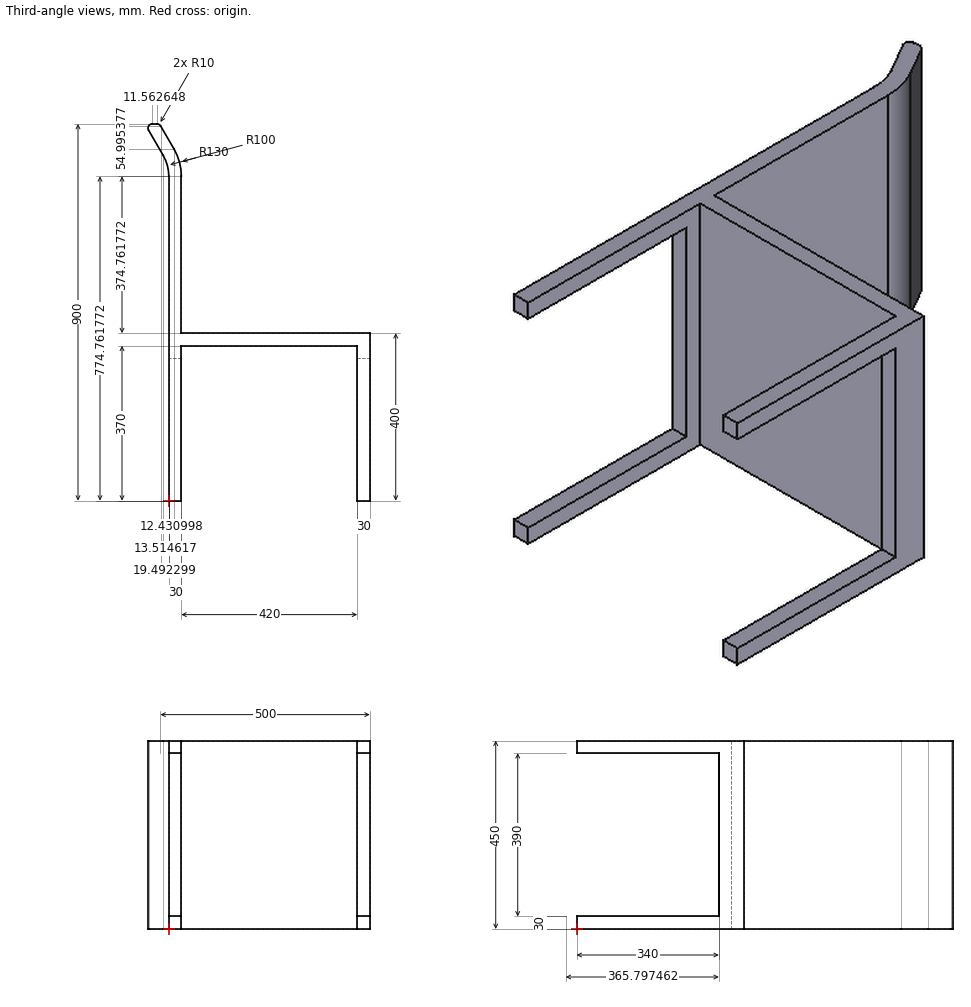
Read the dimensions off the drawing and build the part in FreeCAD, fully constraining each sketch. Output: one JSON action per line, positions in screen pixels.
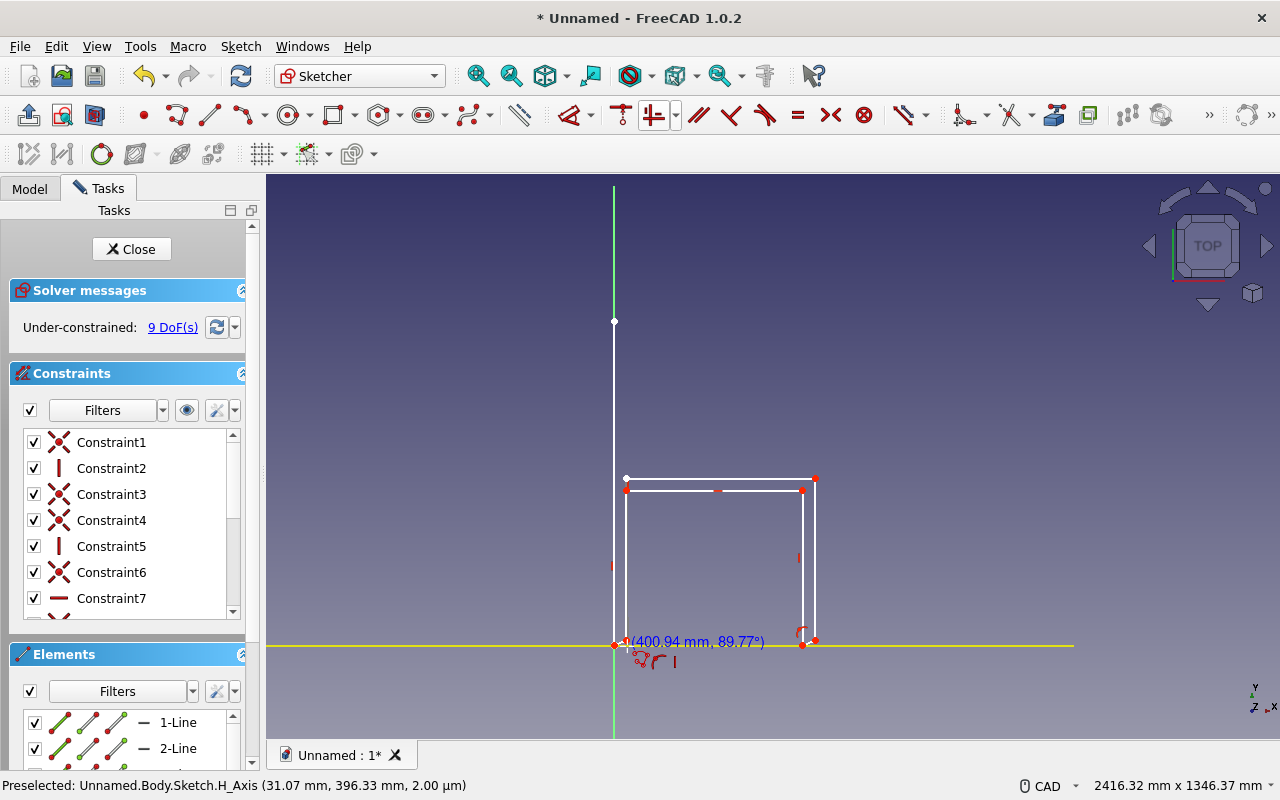
{"action": "scroll", "coordinate": [627, 321], "scroll_direction": "up", "scroll_amount": 2}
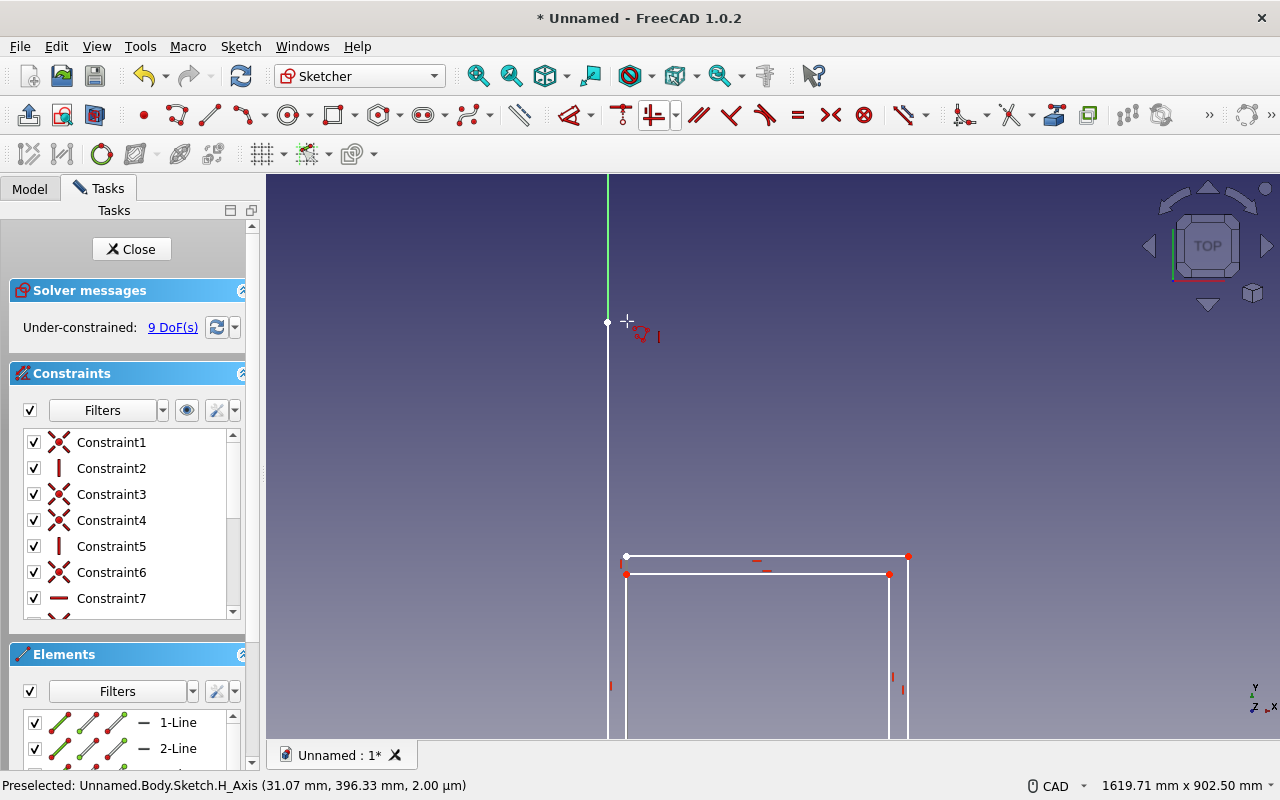
{"action": "left_click", "coordinate": [626, 320]}
{"action": "right_click", "coordinate": [626, 320]}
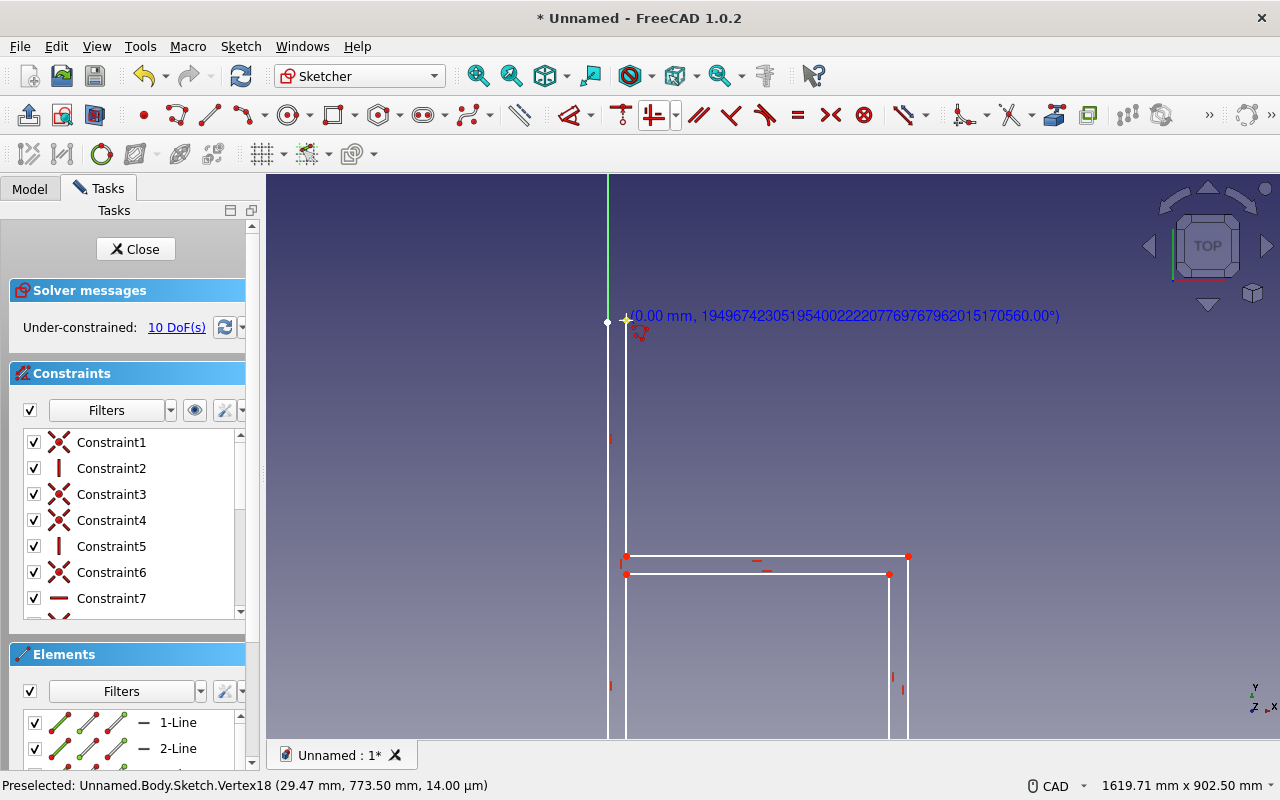
{"action": "key", "text": "g l"}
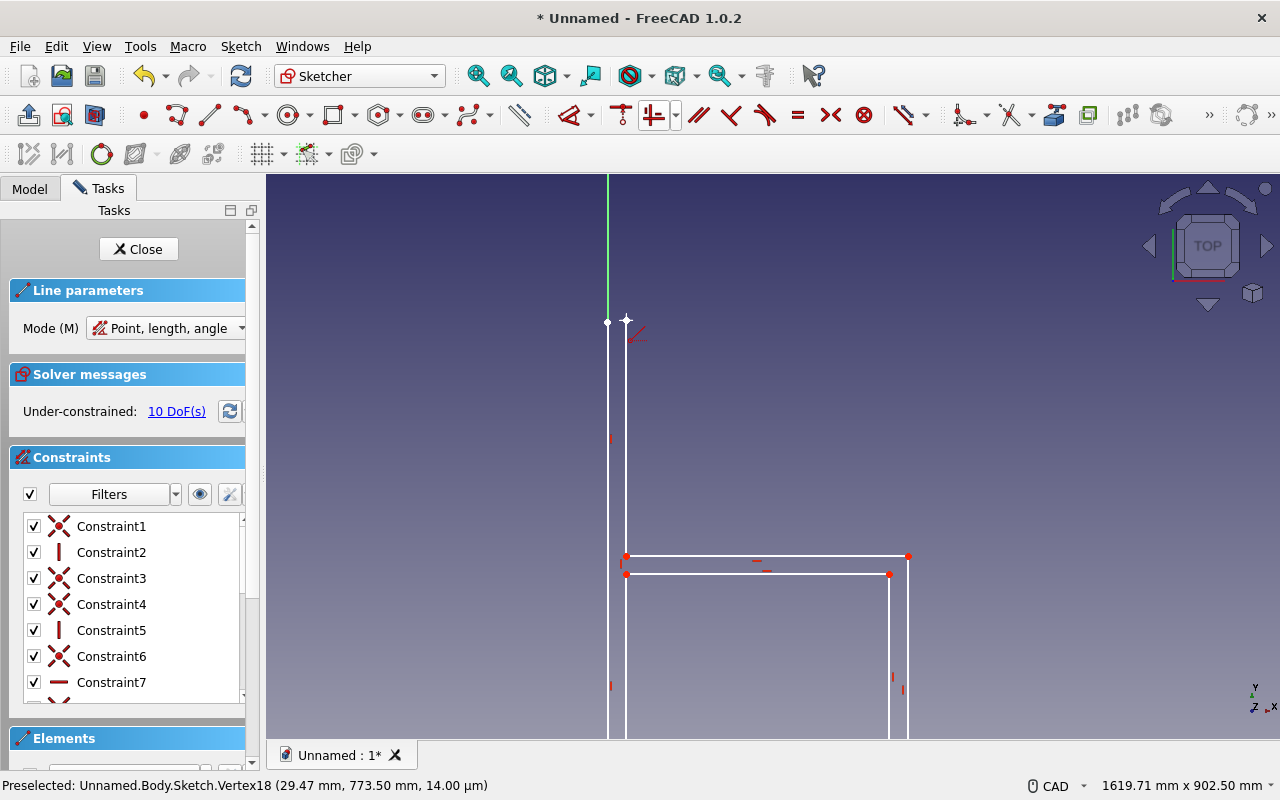
{"action": "scroll", "coordinate": [615, 279], "scroll_direction": "up", "scroll_amount": 4}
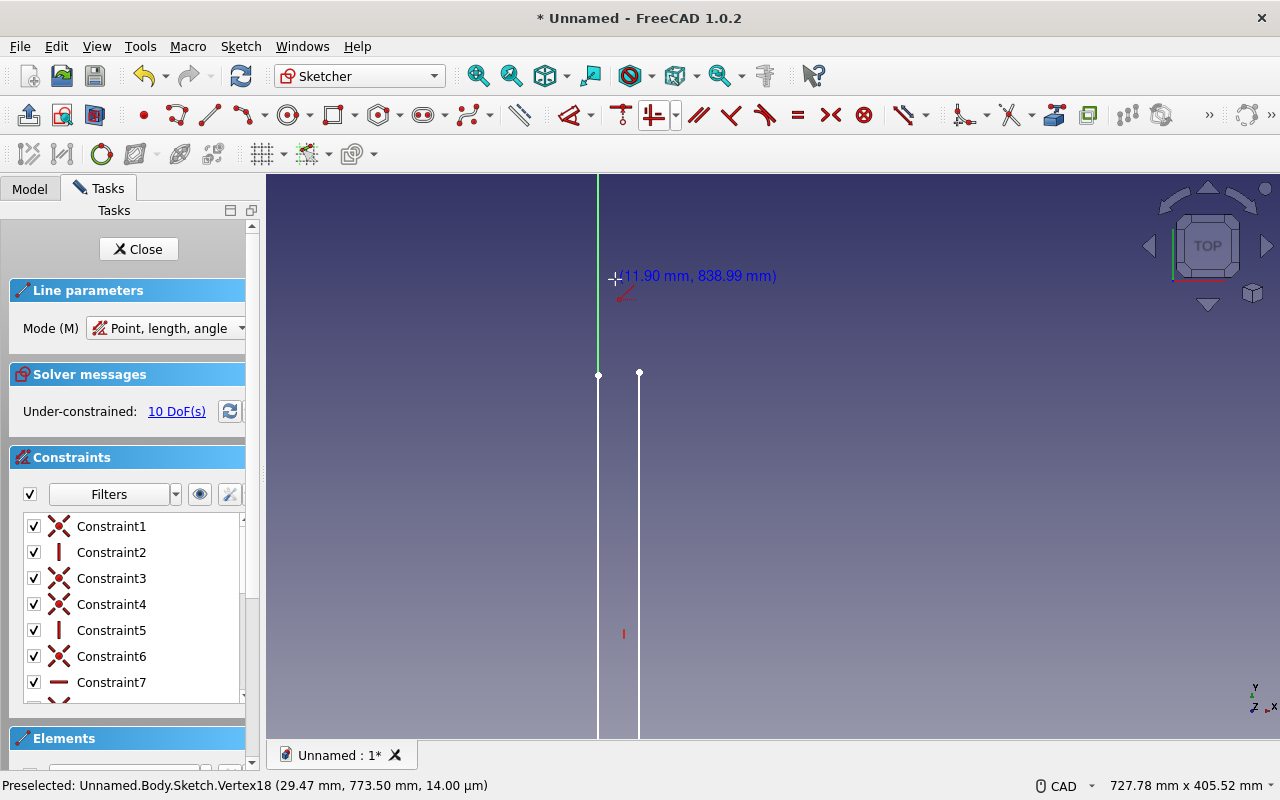
{"action": "left_click", "coordinate": [615, 280]}
{"action": "left_click", "coordinate": [571, 203]}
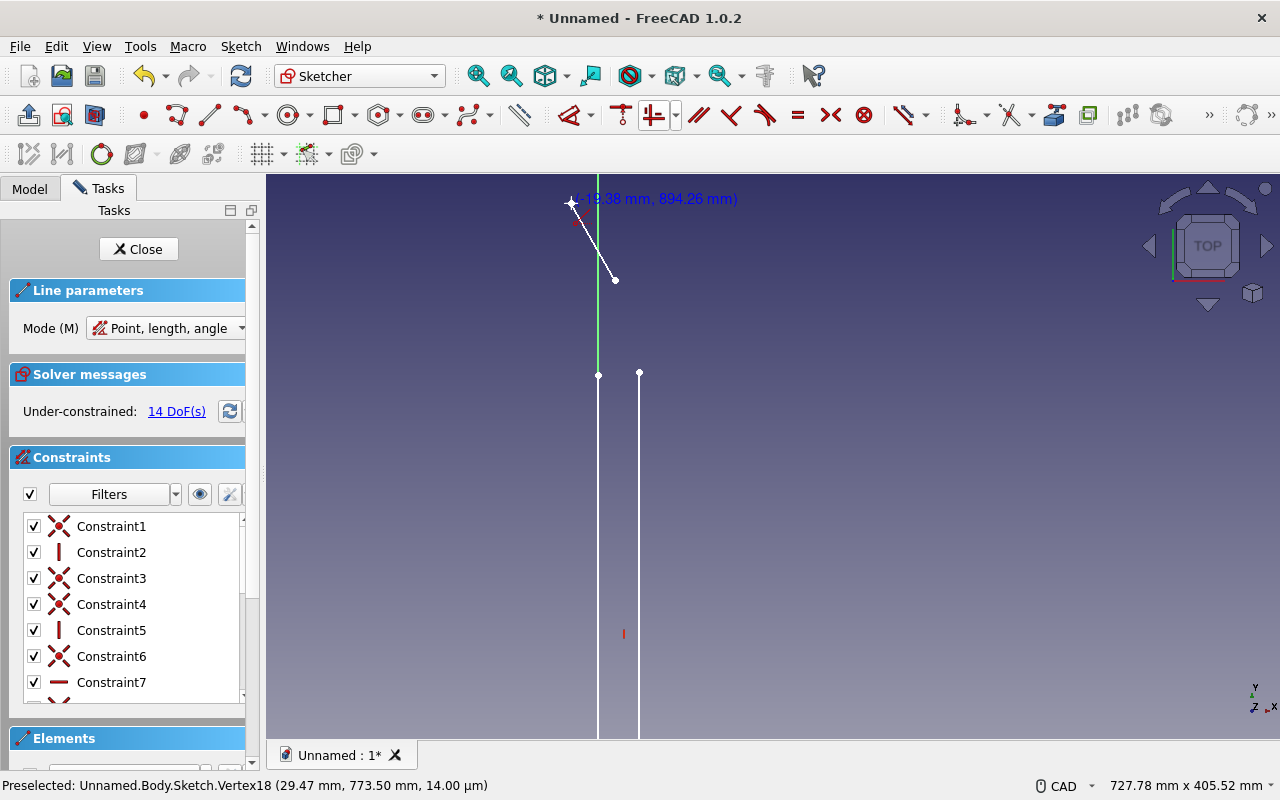
{"action": "scroll", "coordinate": [621, 299], "scroll_direction": "down", "scroll_amount": 6}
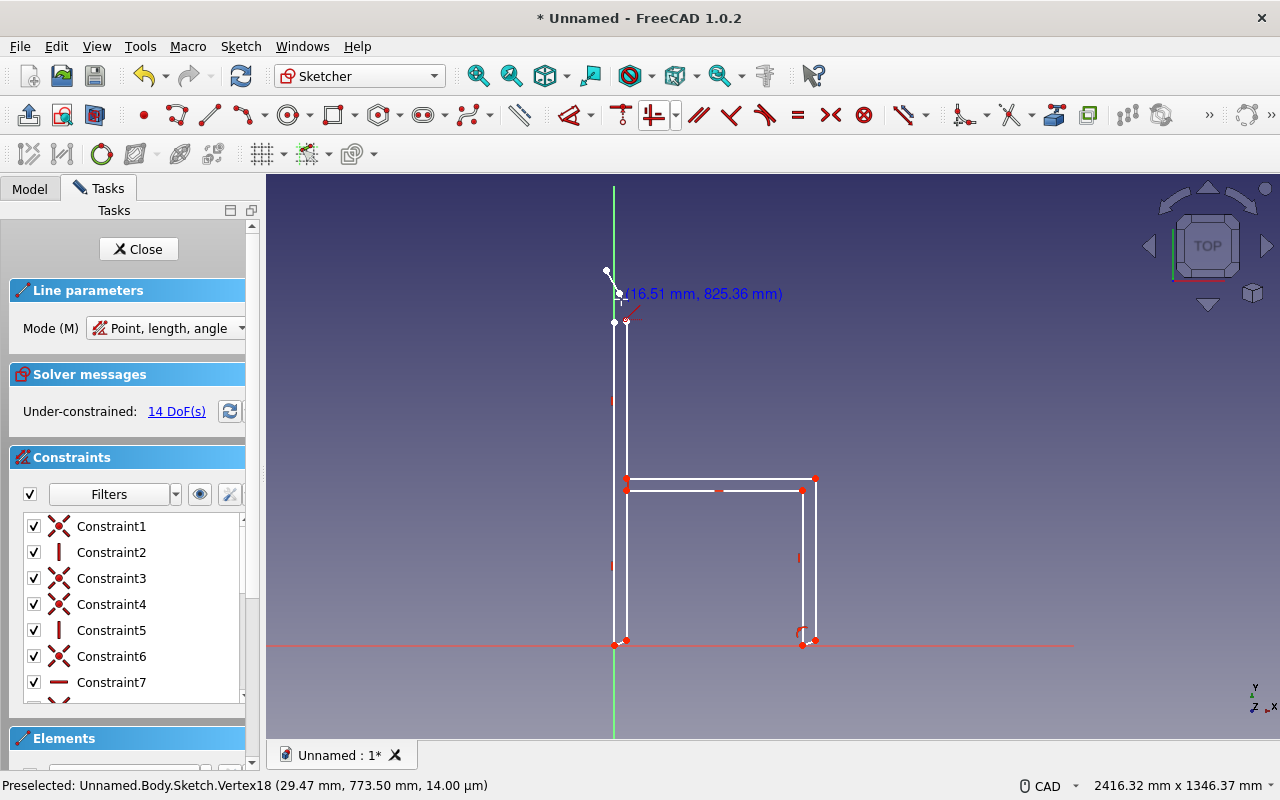
{"action": "scroll", "coordinate": [603, 268], "scroll_direction": "up", "scroll_amount": 7}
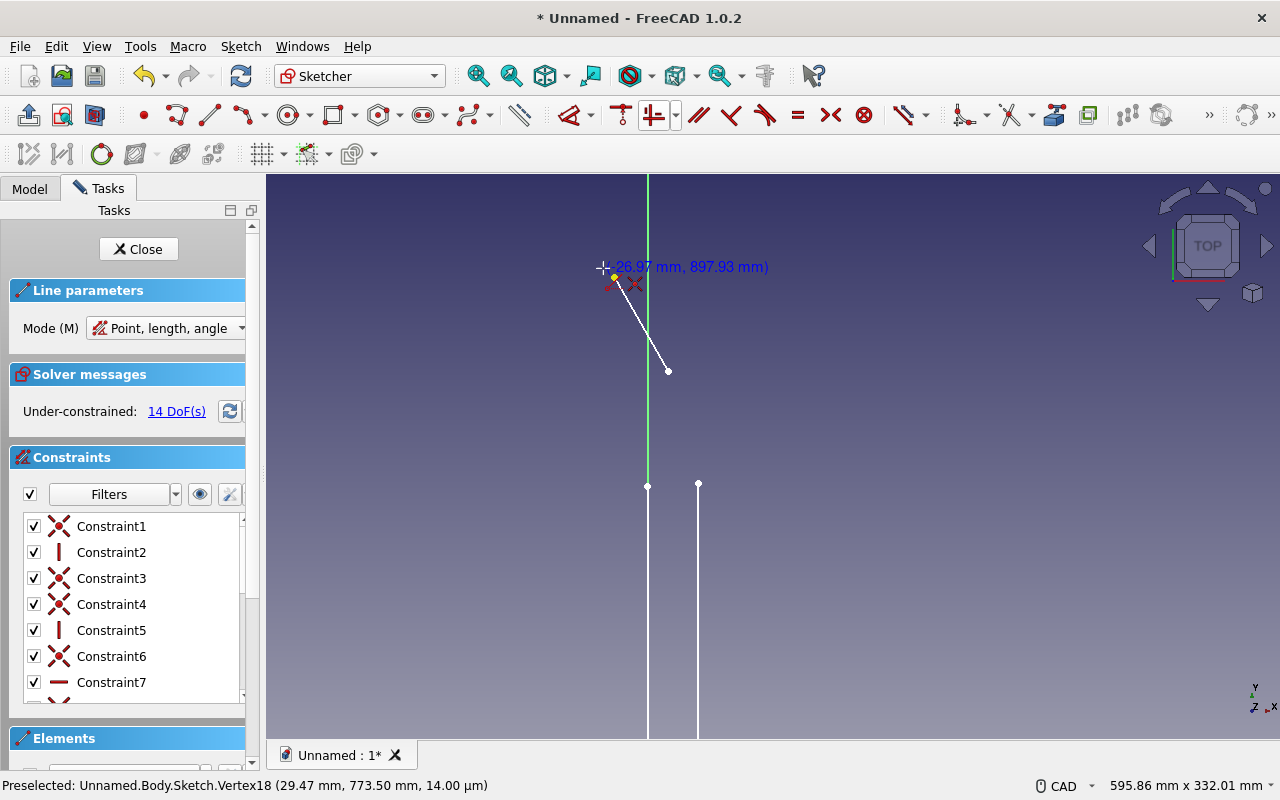
{"action": "left_click", "coordinate": [600, 268]}
{"action": "left_click", "coordinate": [580, 268]}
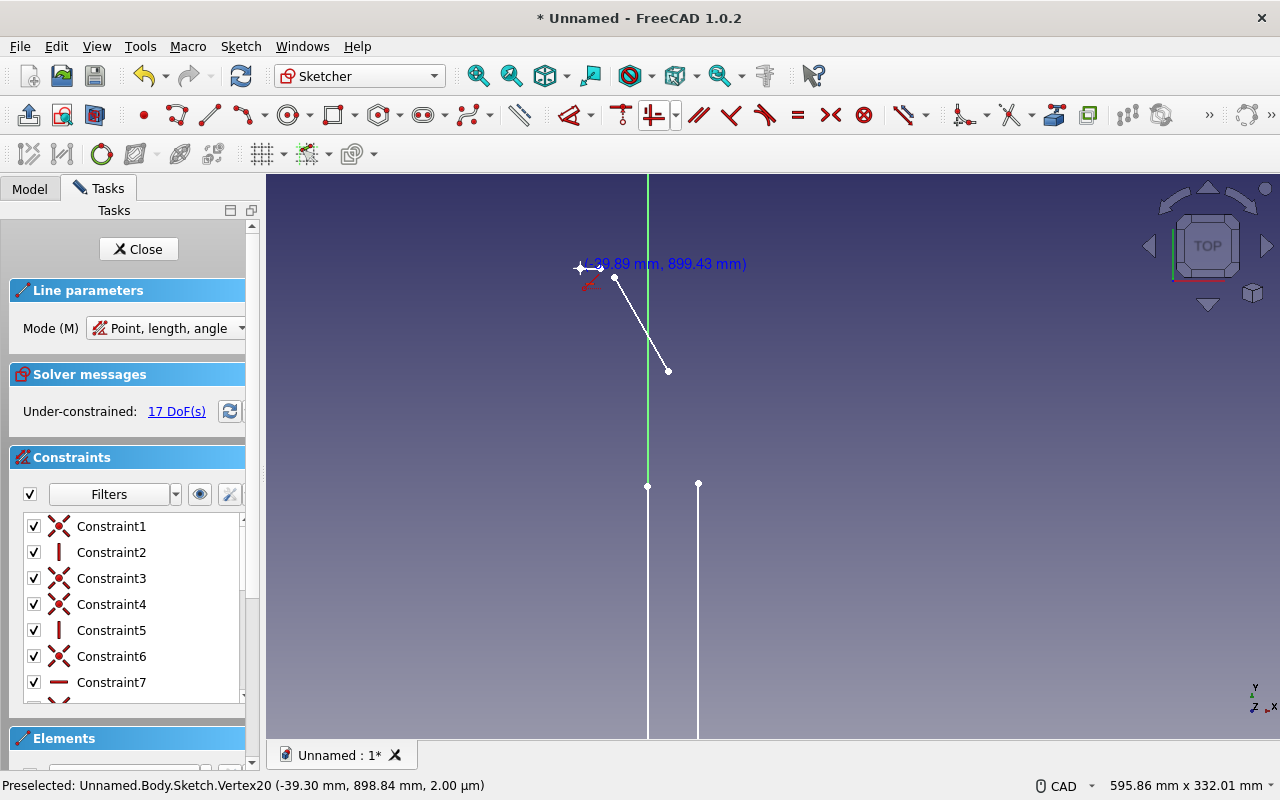
{"action": "left_click", "coordinate": [566, 294]}
{"action": "left_click", "coordinate": [625, 396]}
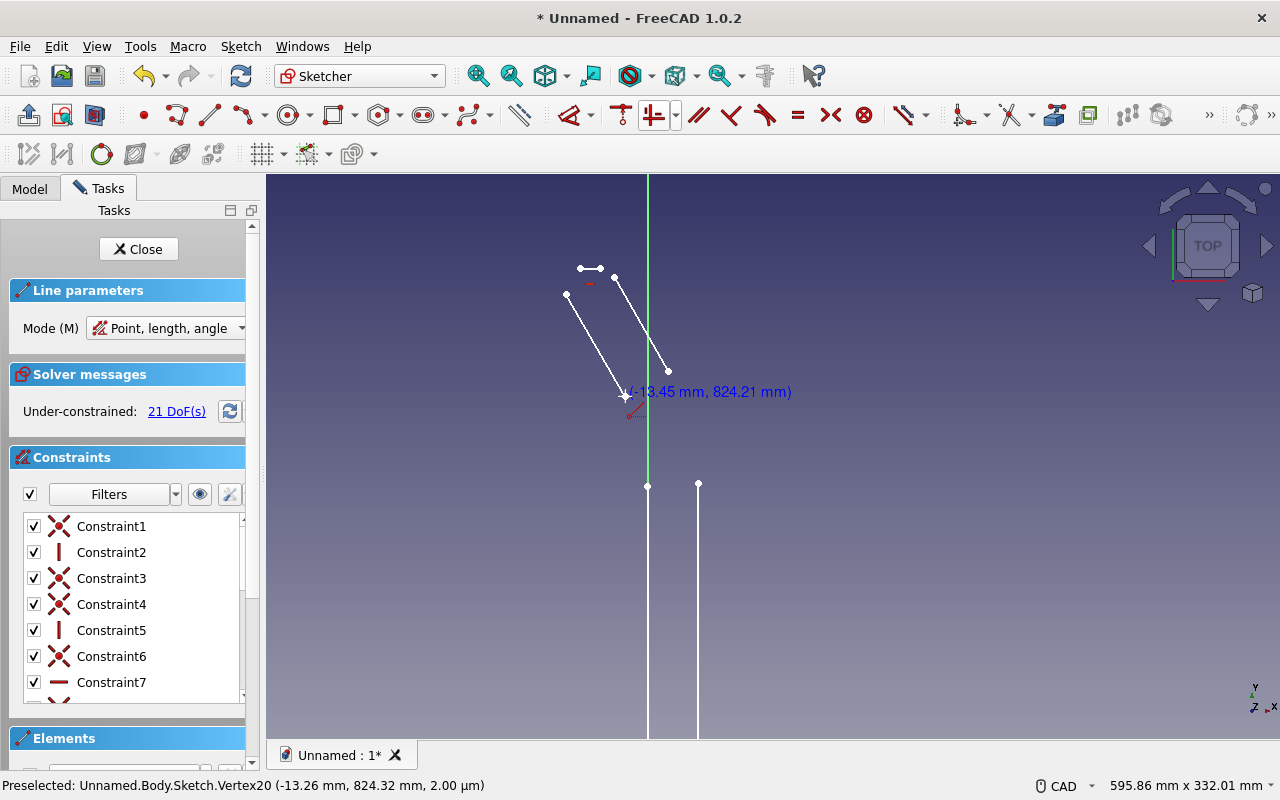
{"action": "left_click", "coordinate": [242, 116]}